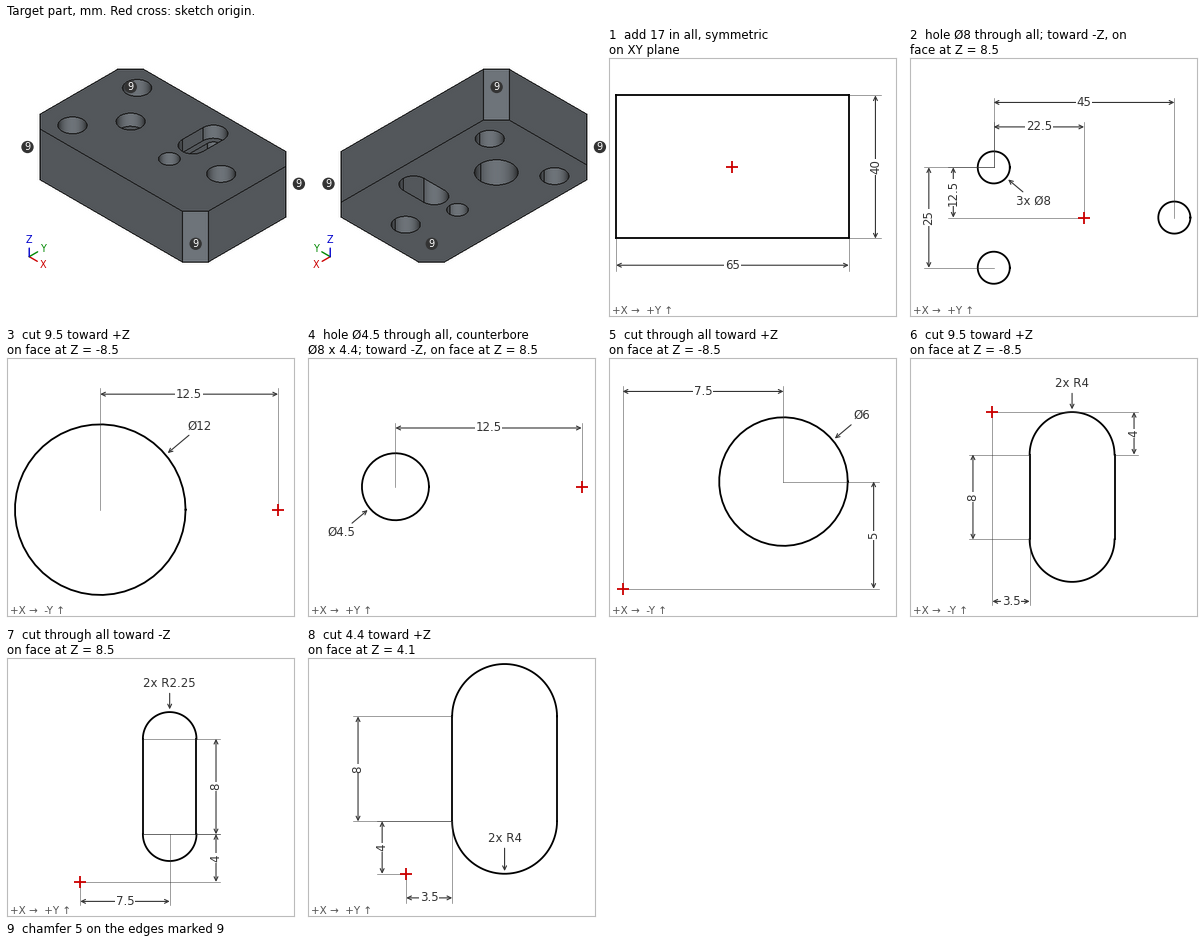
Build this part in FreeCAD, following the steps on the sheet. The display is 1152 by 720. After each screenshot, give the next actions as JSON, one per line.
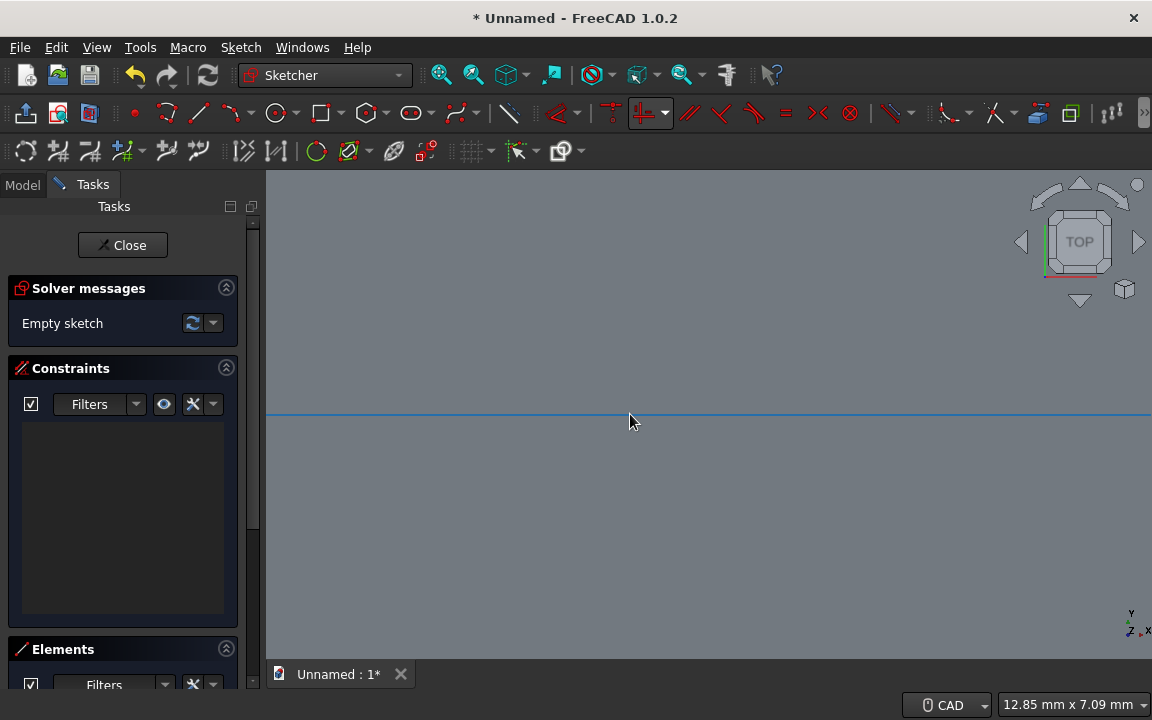
{"action": "left_click", "coordinate": [276, 114]}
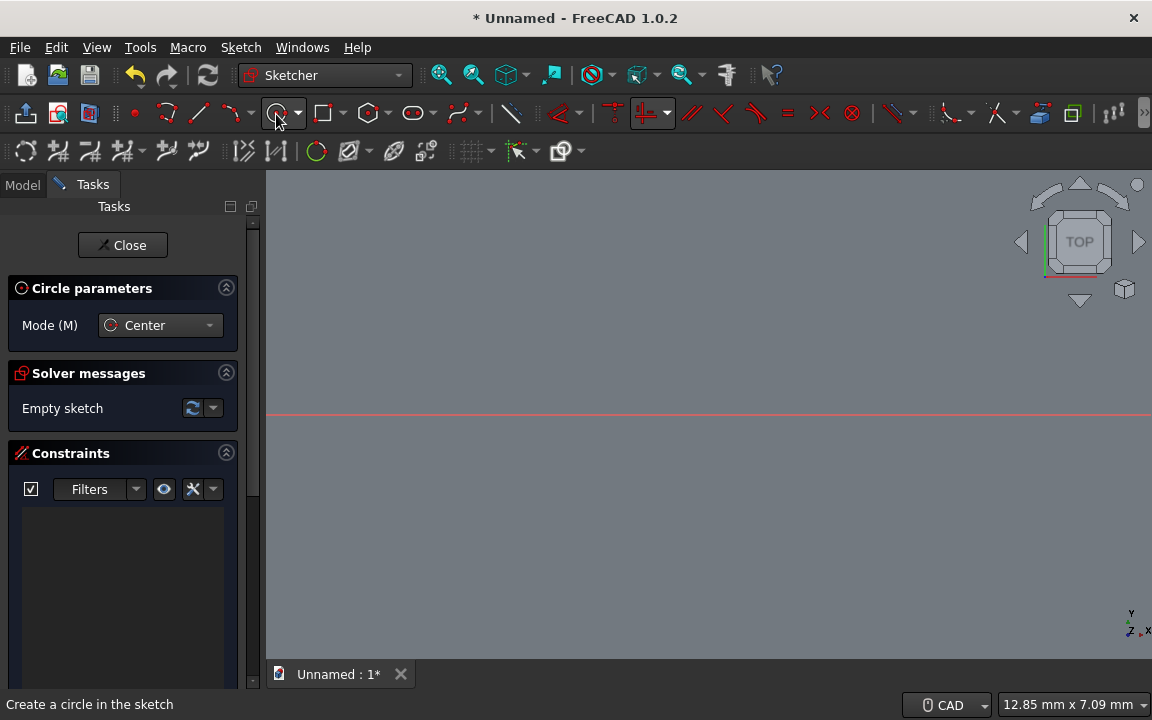
{"action": "left_click", "coordinate": [635, 414]}
{"action": "left_click", "coordinate": [745, 305]}
{"action": "key", "text": "Escape"}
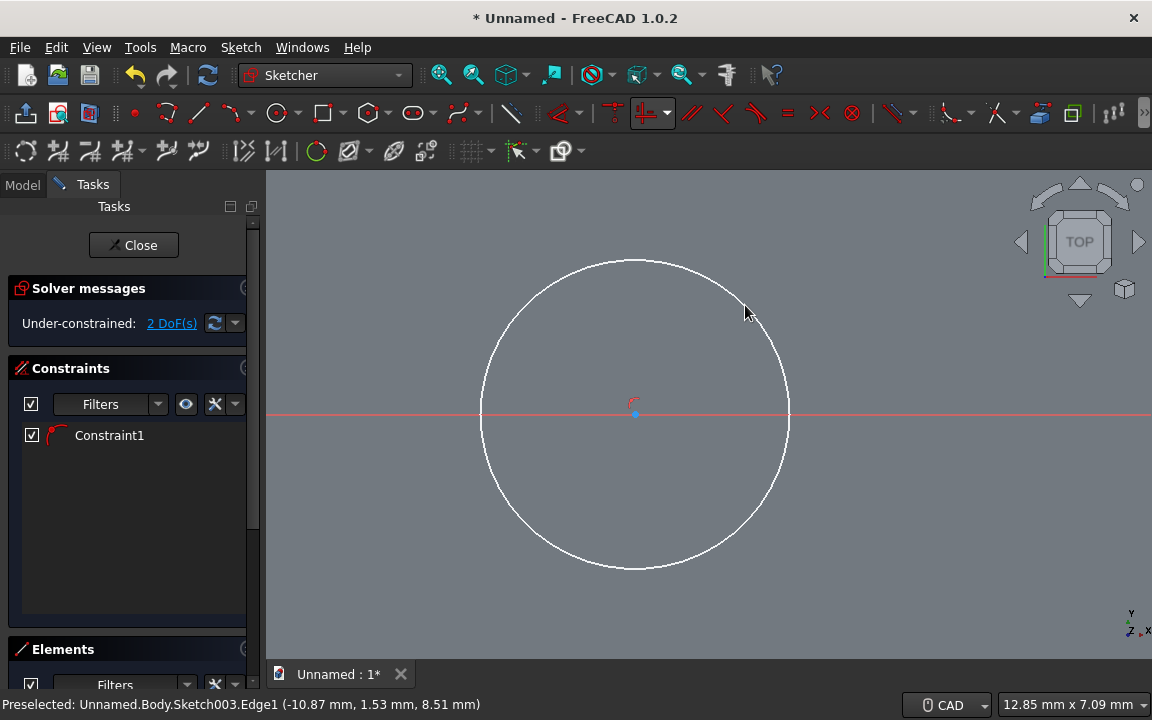
{"action": "left_click", "coordinate": [558, 114]}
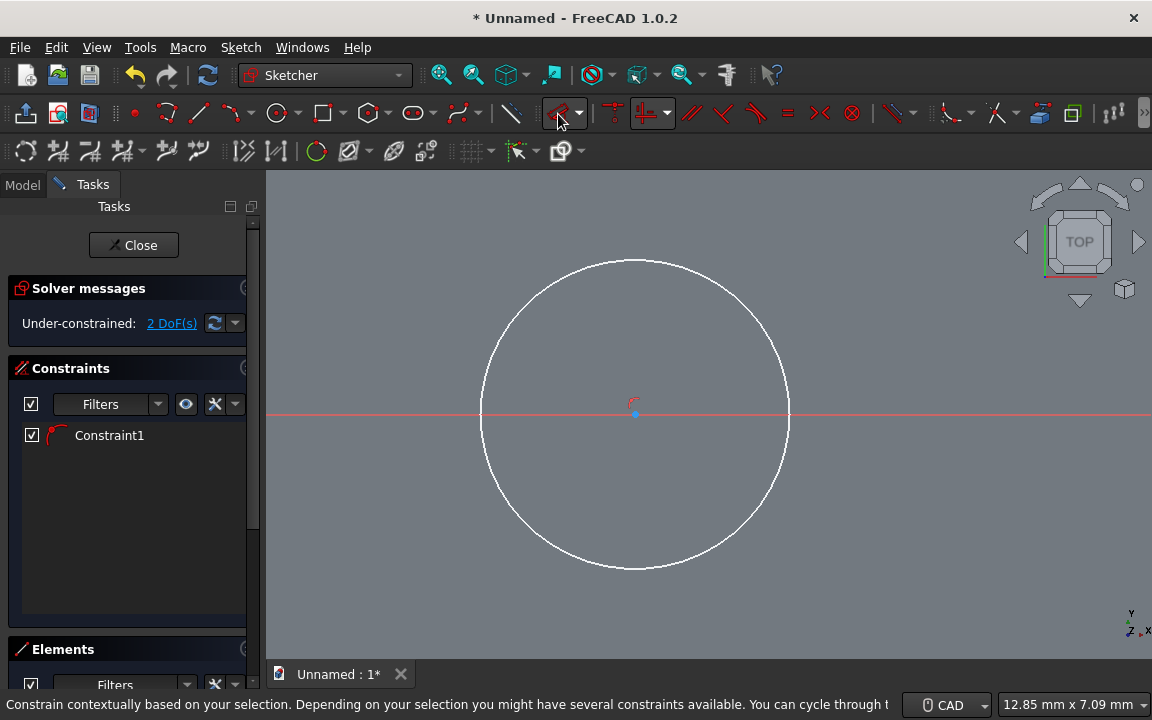
{"action": "left_click", "coordinate": [744, 305]}
{"action": "left_click", "coordinate": [767, 282]}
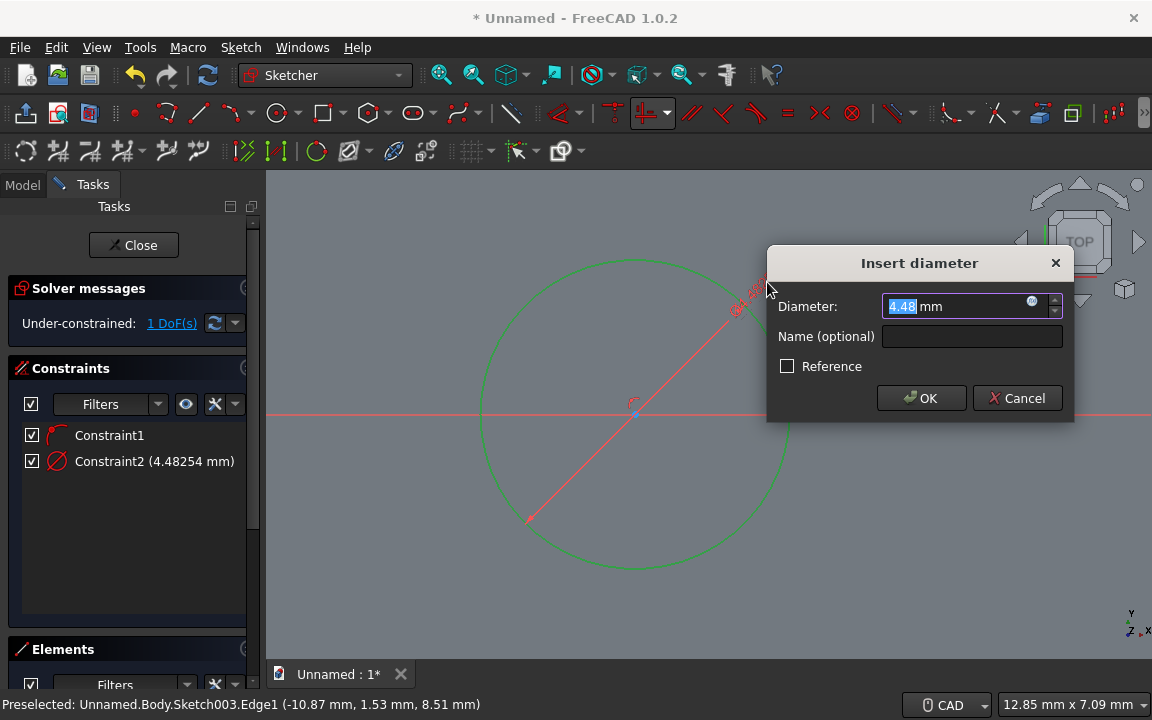
{"action": "type", "text": "4.5"}
{"action": "key", "text": "Return"}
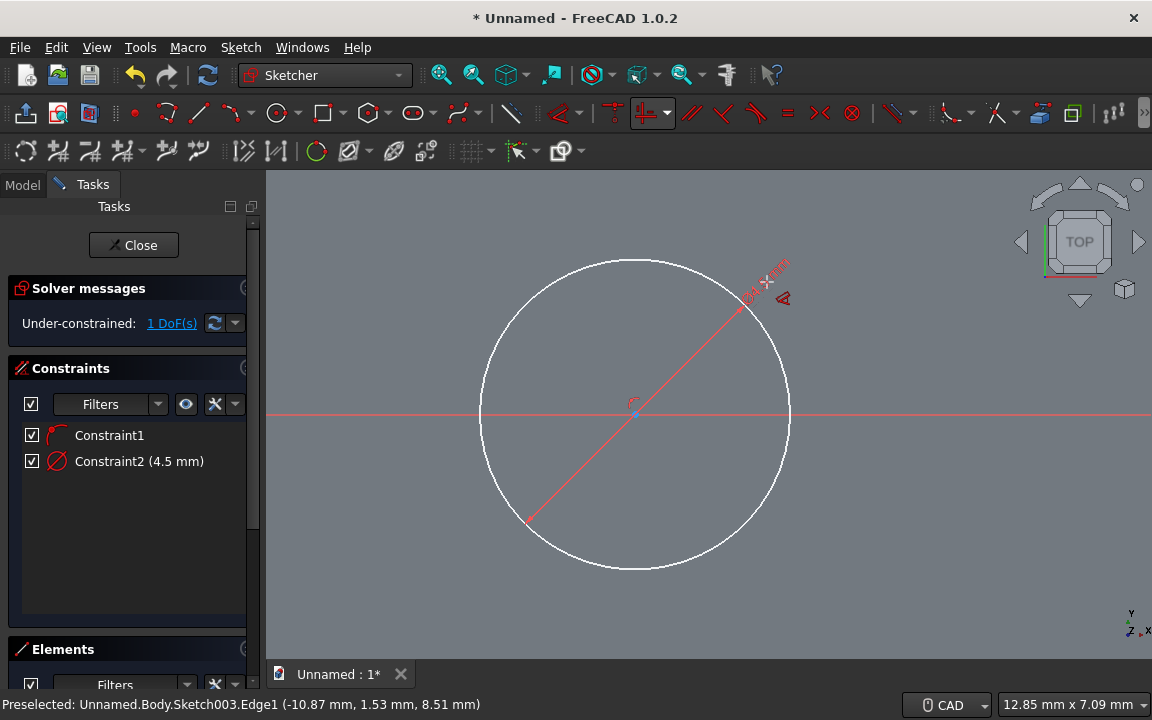
{"action": "left_click", "coordinate": [635, 414]}
{"action": "left_click", "coordinate": [811, 448]}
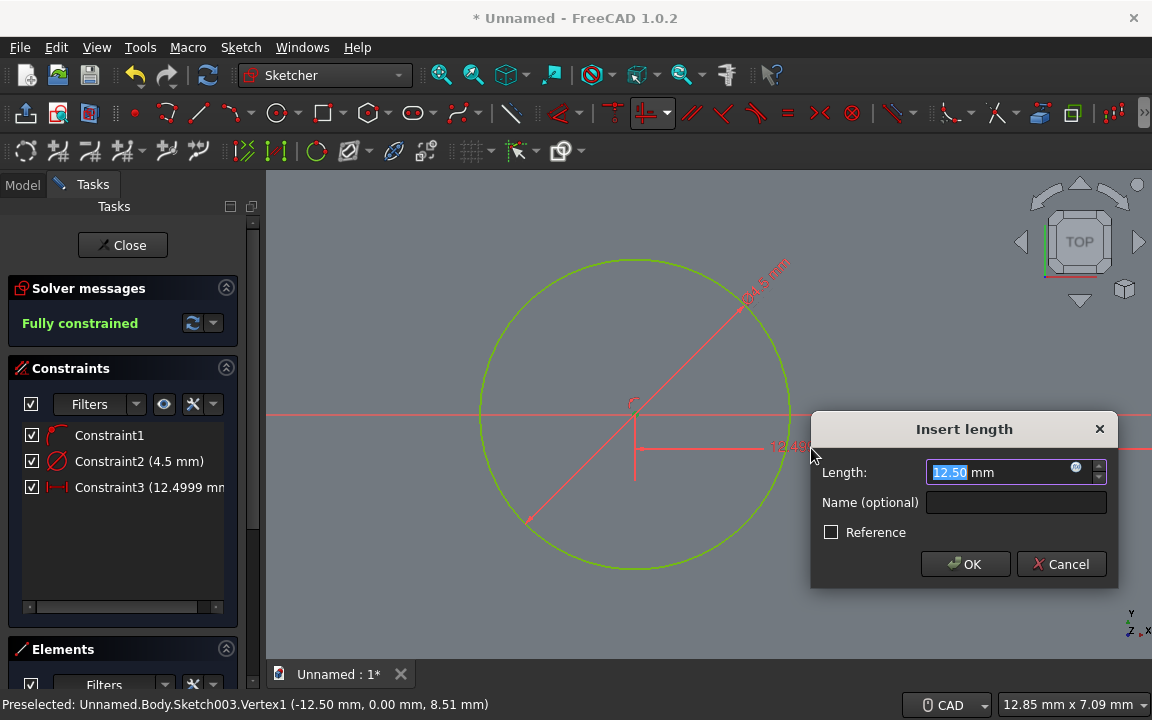
{"action": "type", "text": "12.5"}
{"action": "key", "text": "Return"}
{"action": "key", "text": "Escape"}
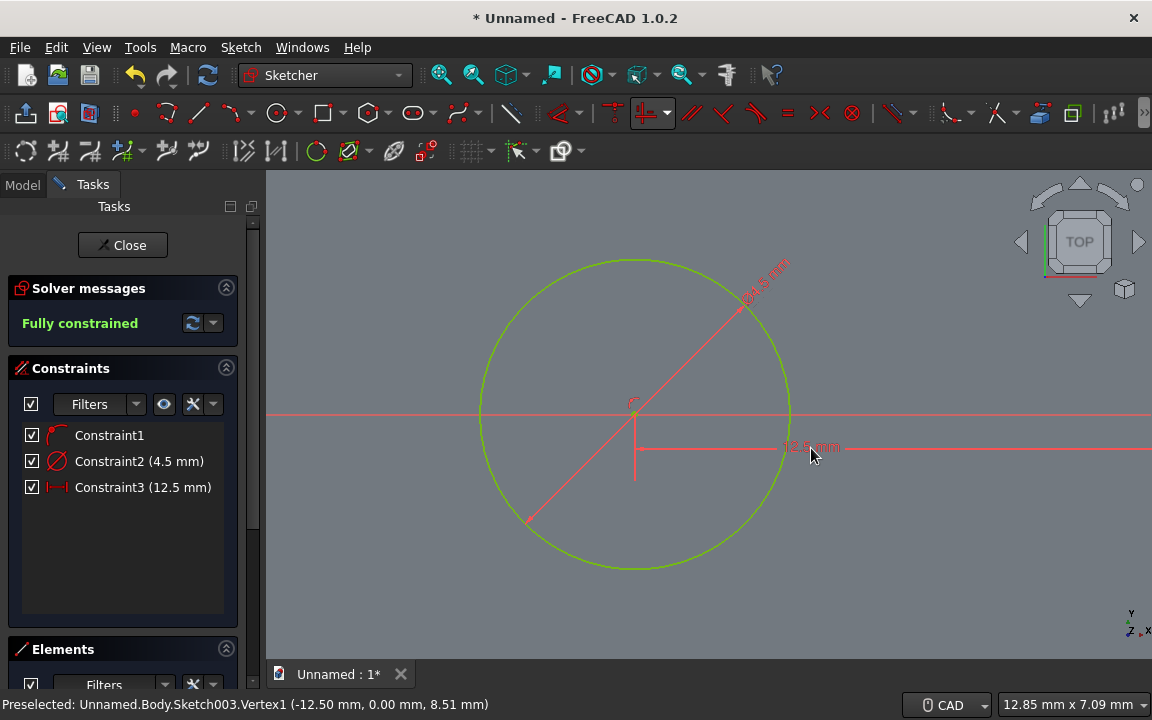
{"action": "left_click", "coordinate": [123, 245]}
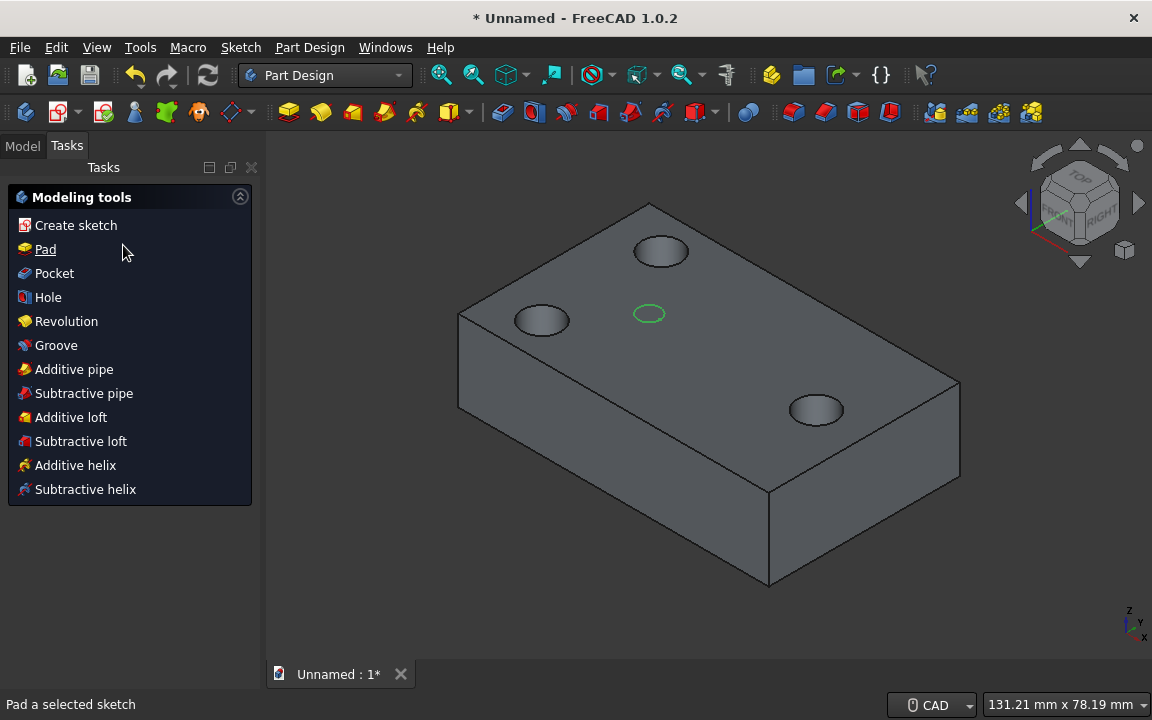
{"action": "left_click", "coordinate": [536, 112]}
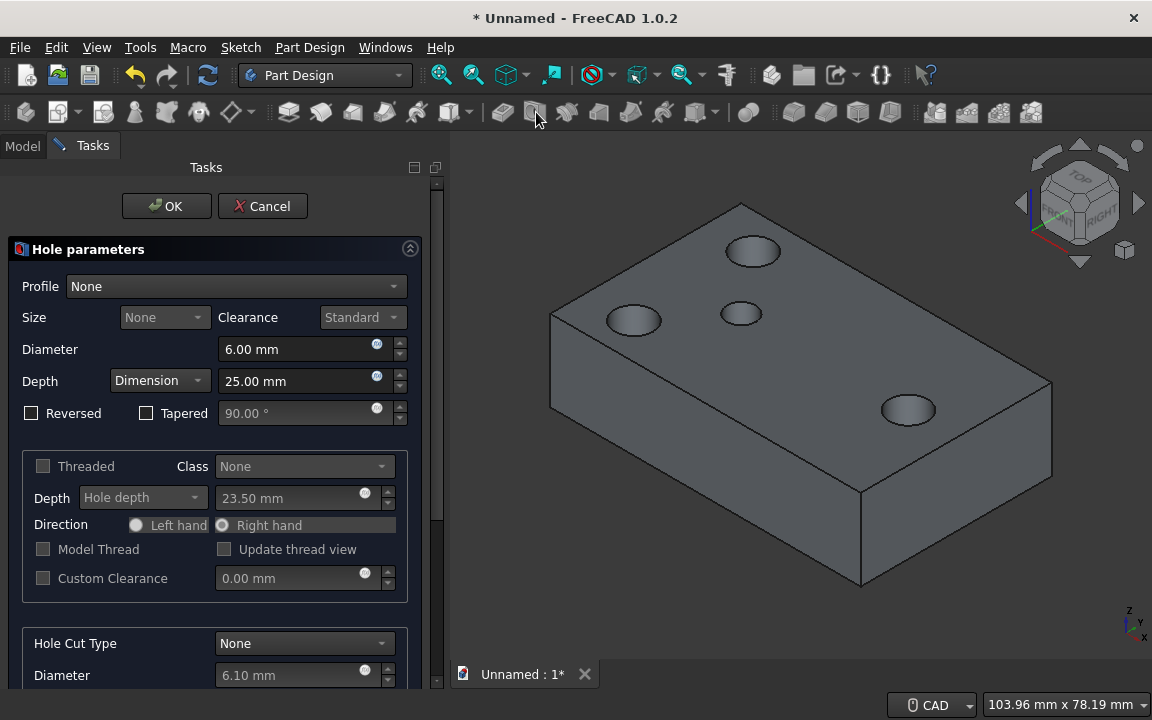
{"action": "triple_click", "coordinate": [305, 349]}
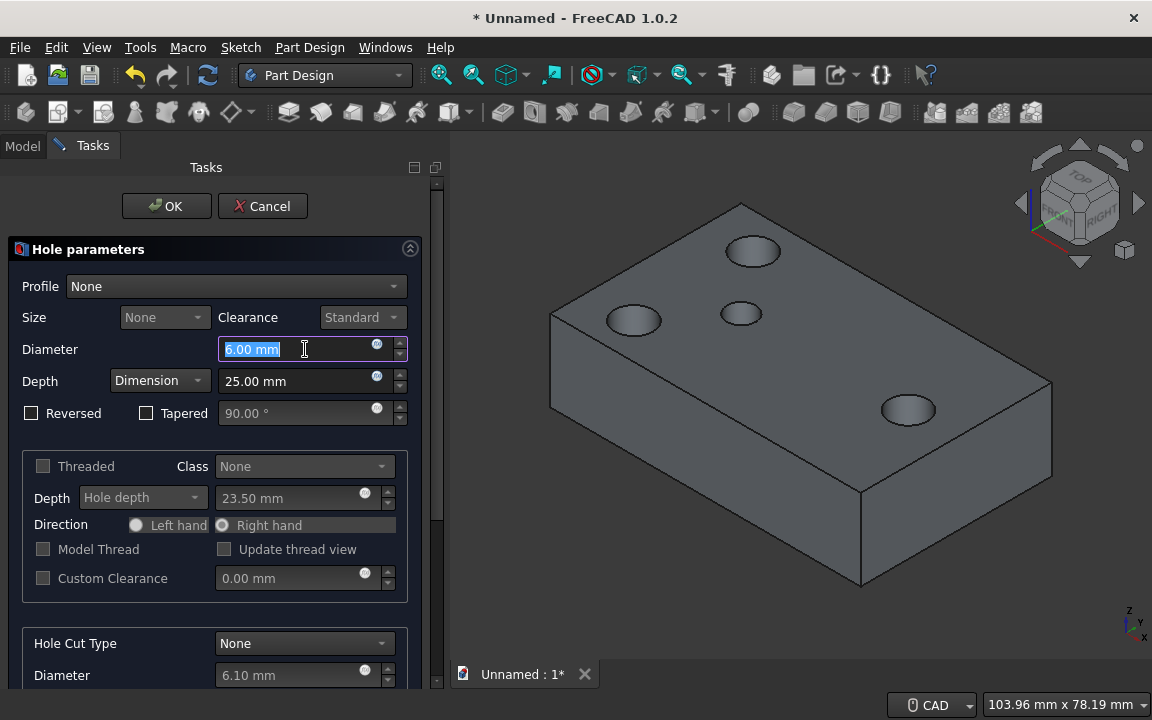
{"action": "type", "text": "4.5"}
{"action": "key", "text": "Tab"}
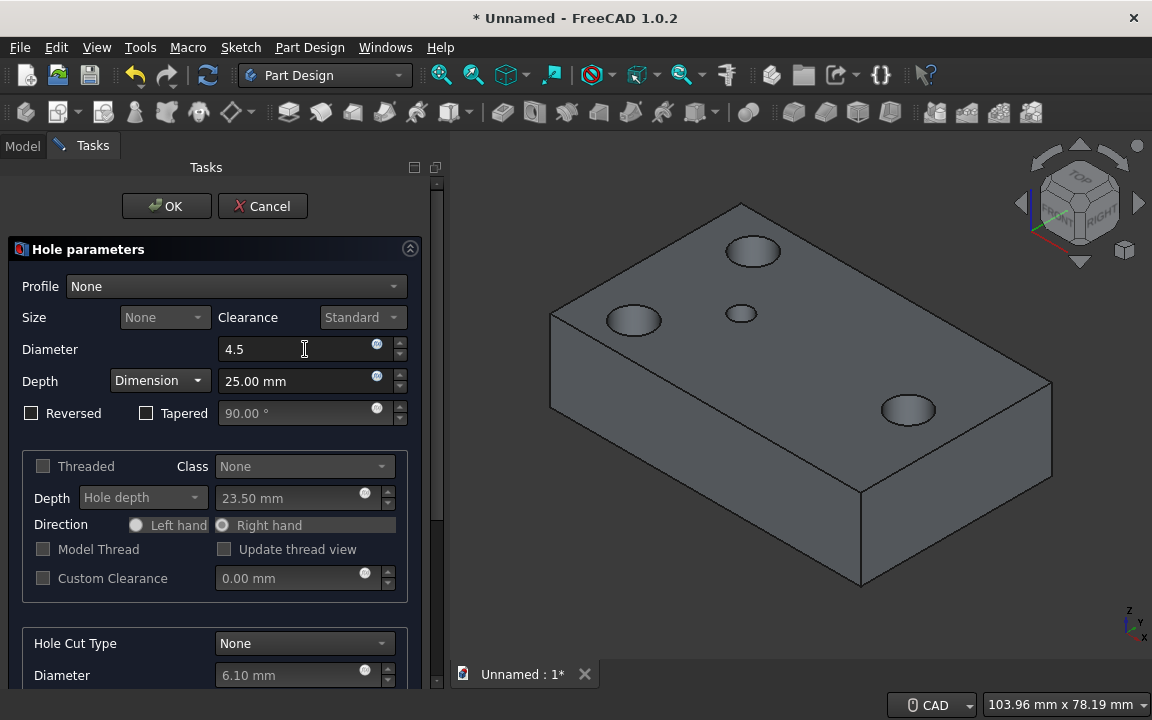
{"action": "left_click", "coordinate": [161, 380]}